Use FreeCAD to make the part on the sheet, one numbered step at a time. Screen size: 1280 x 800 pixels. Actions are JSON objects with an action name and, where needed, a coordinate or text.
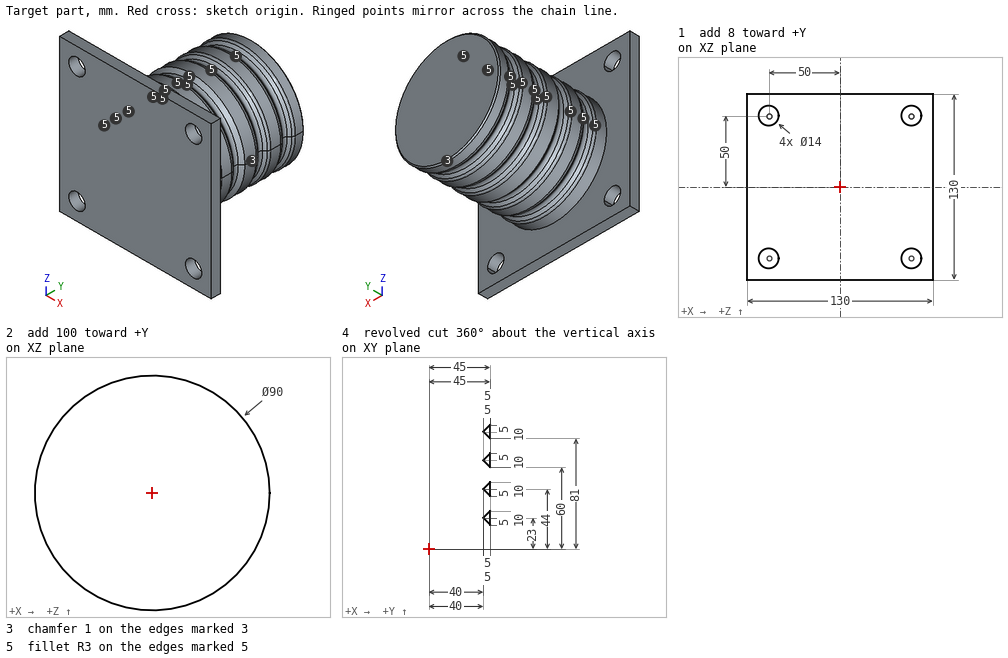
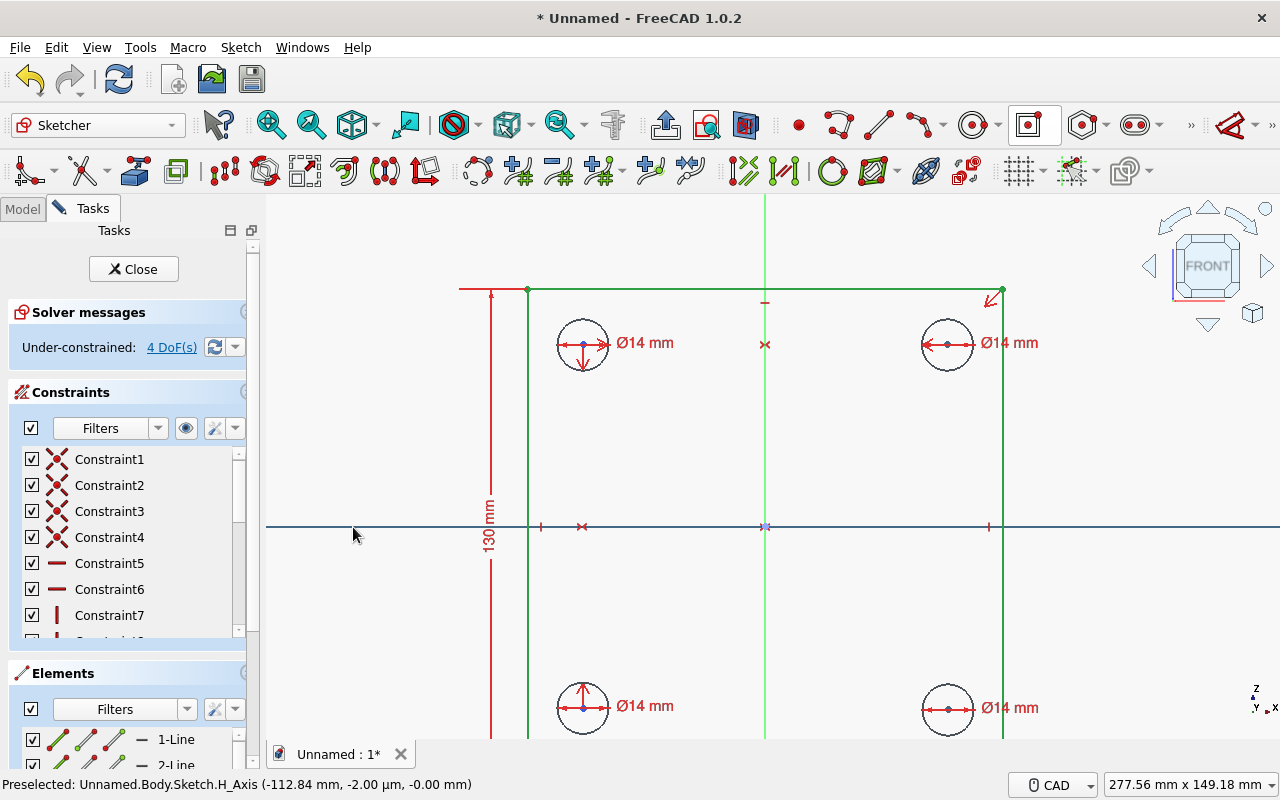
{"action": "key", "text": "s"}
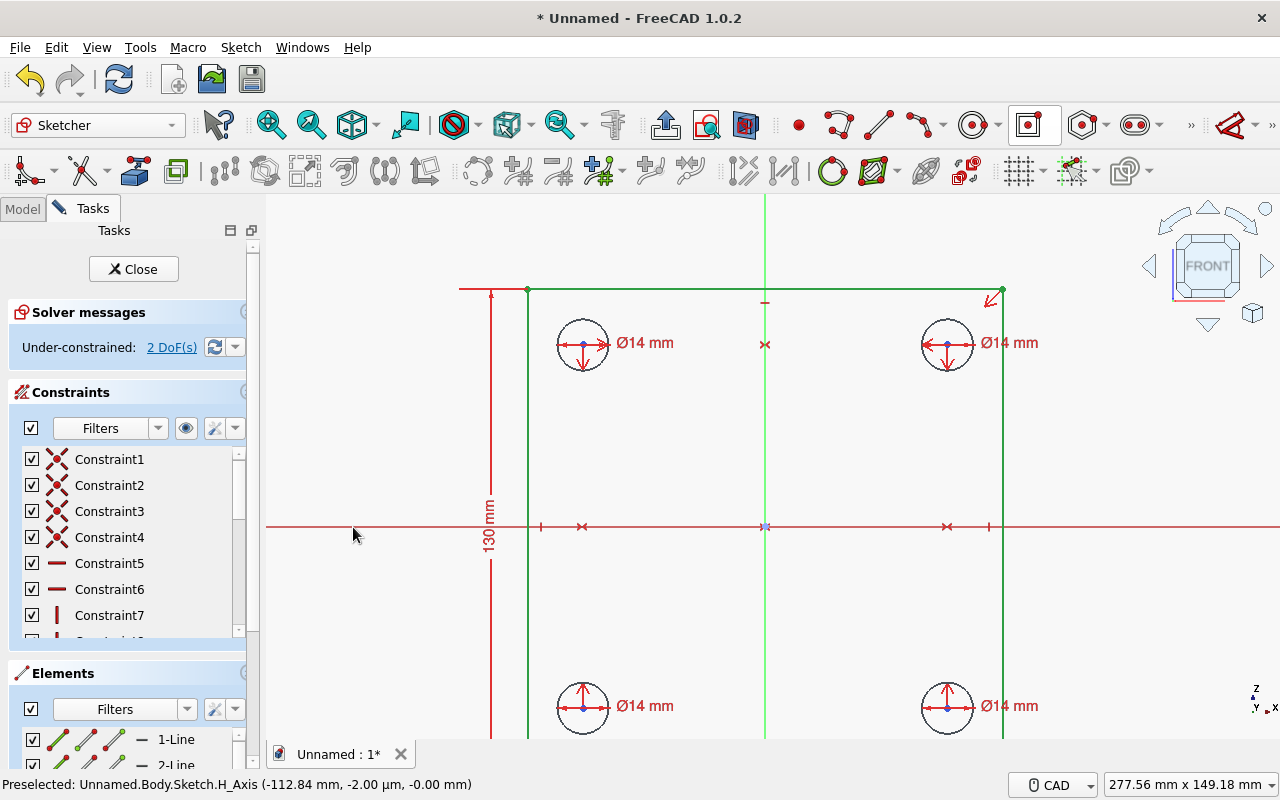
{"action": "left_click", "coordinate": [583, 345]}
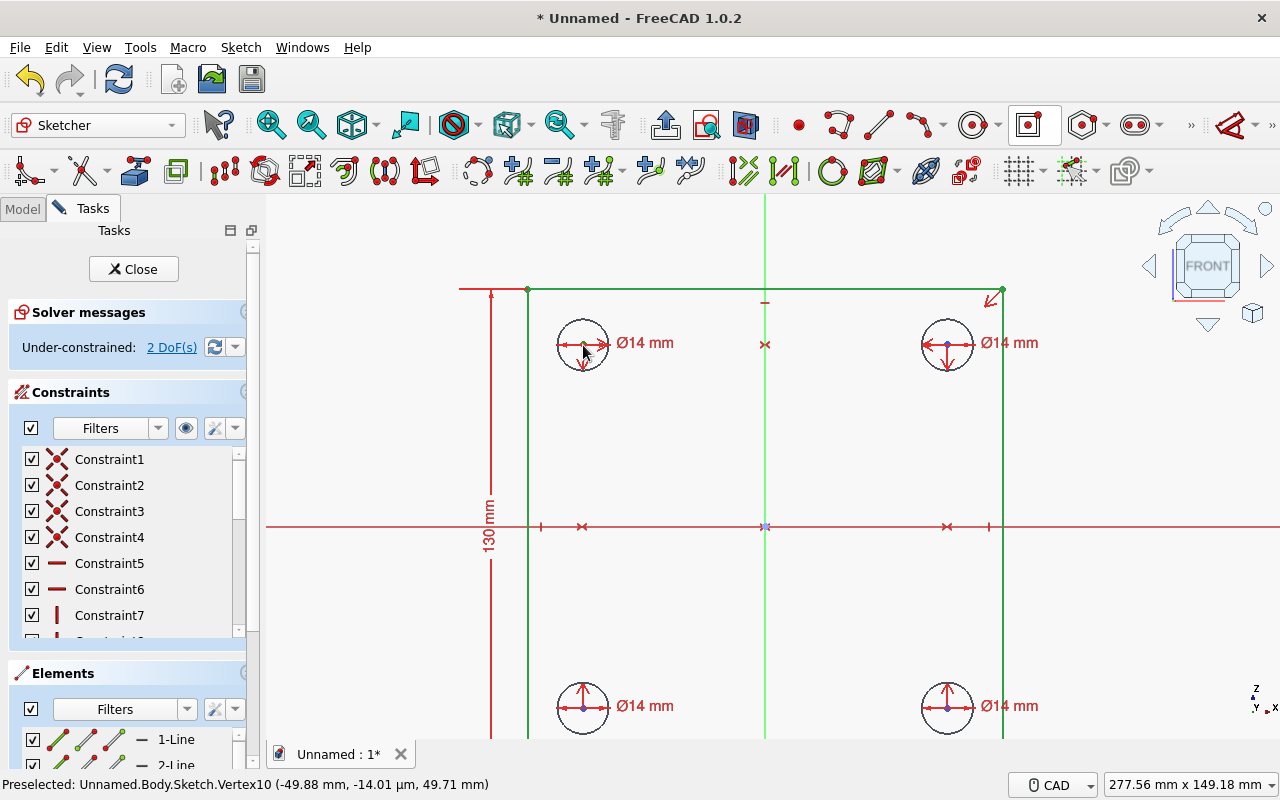
{"action": "left_click", "coordinate": [1258, 126]}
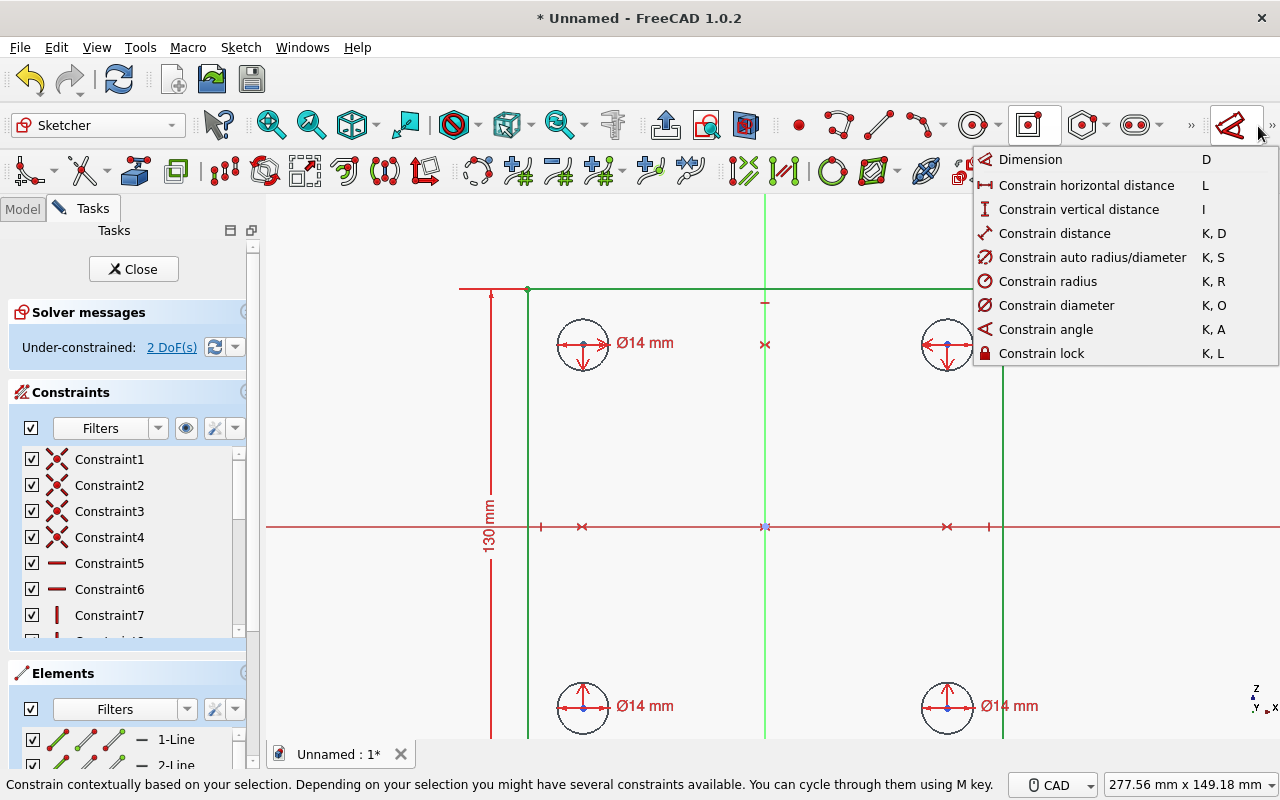
{"action": "left_click", "coordinate": [1126, 185]}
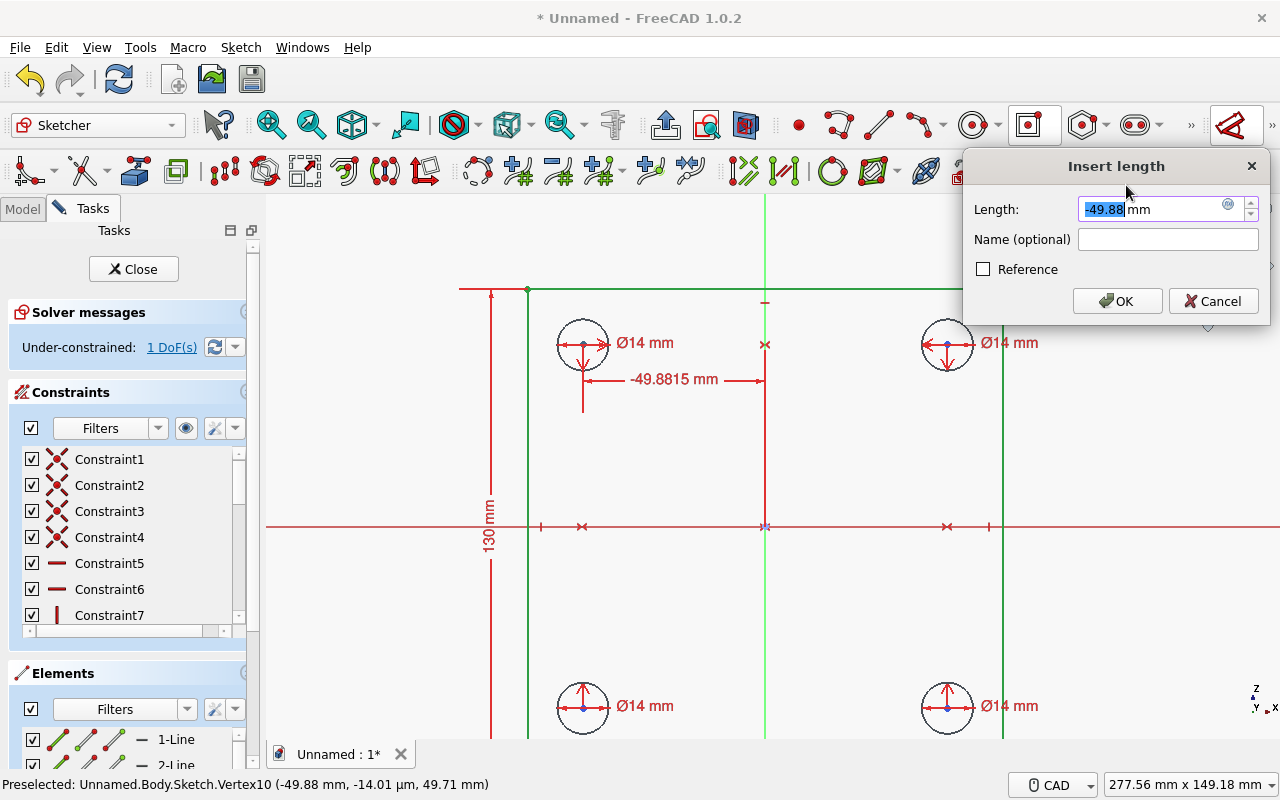
{"action": "type", "text": "-50"}
{"action": "key", "text": "Return"}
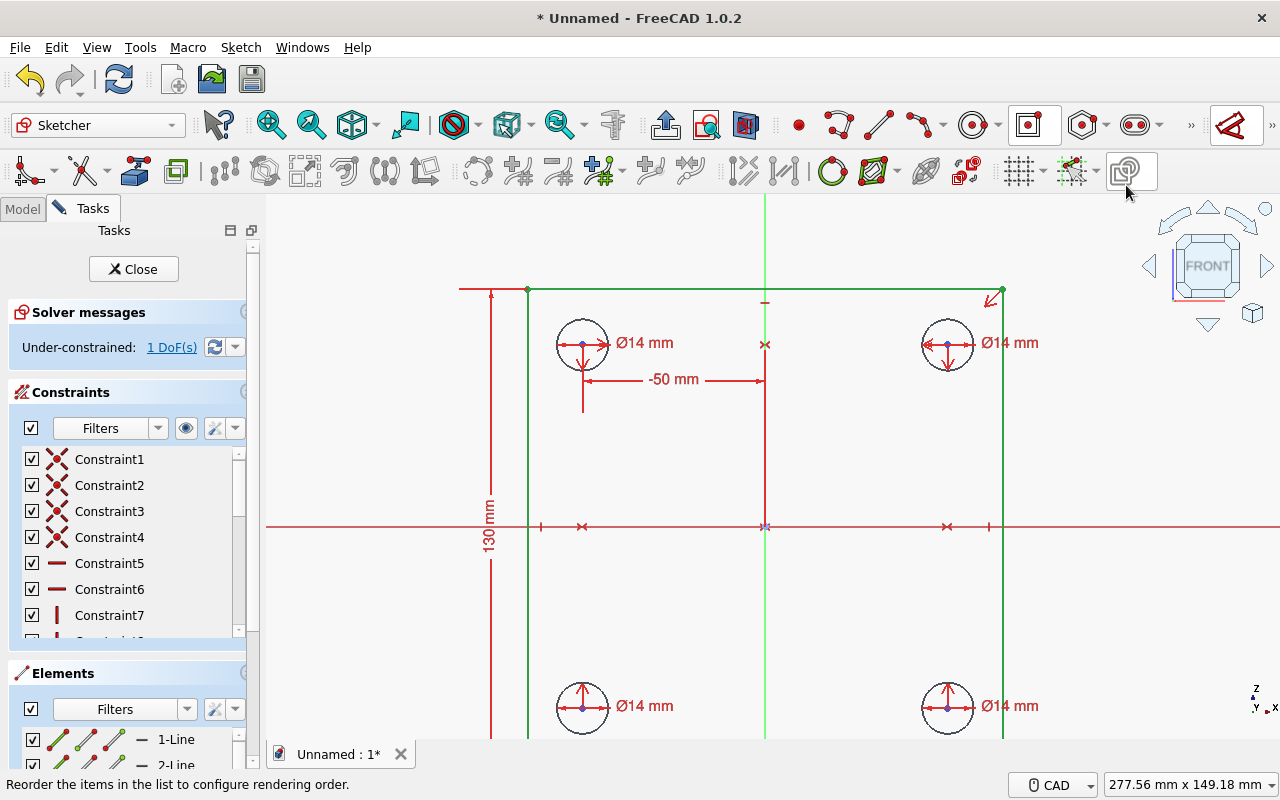
{"action": "left_click", "coordinate": [583, 345]}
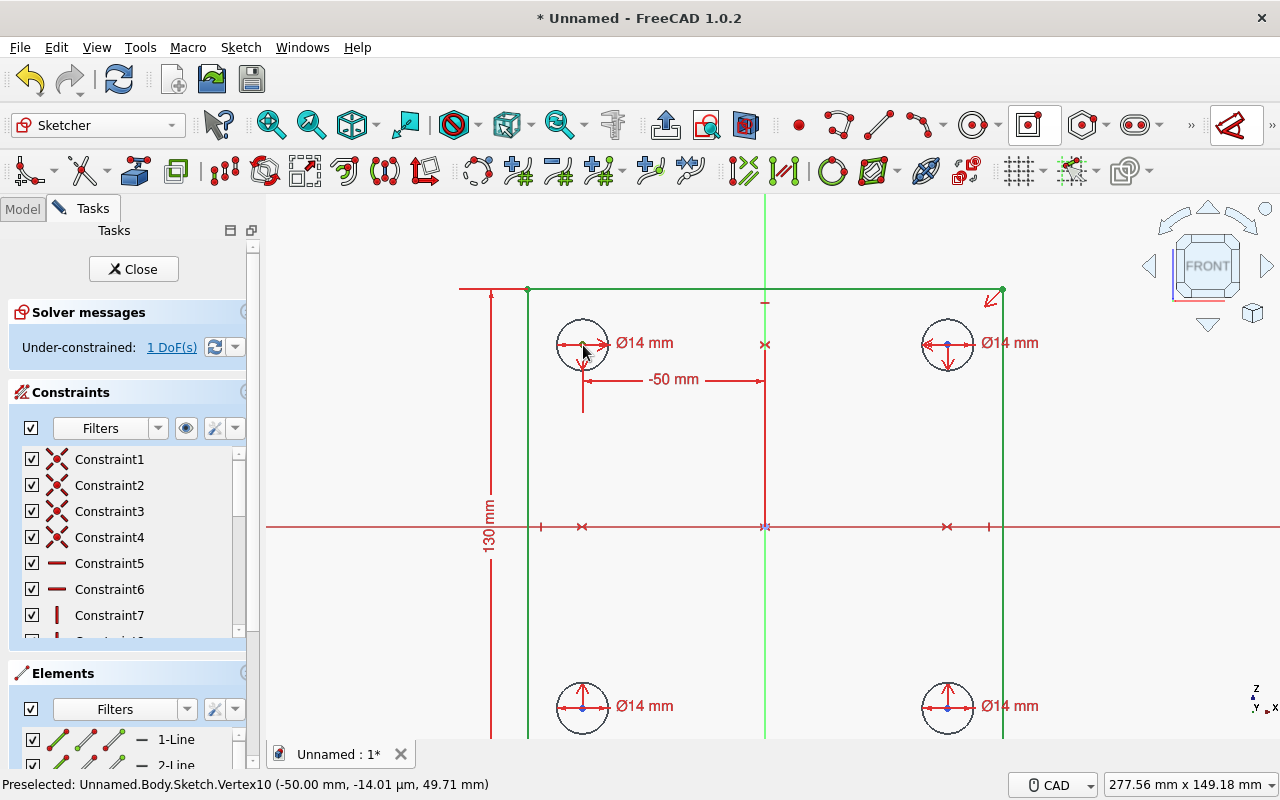
{"action": "left_click", "coordinate": [1258, 126]}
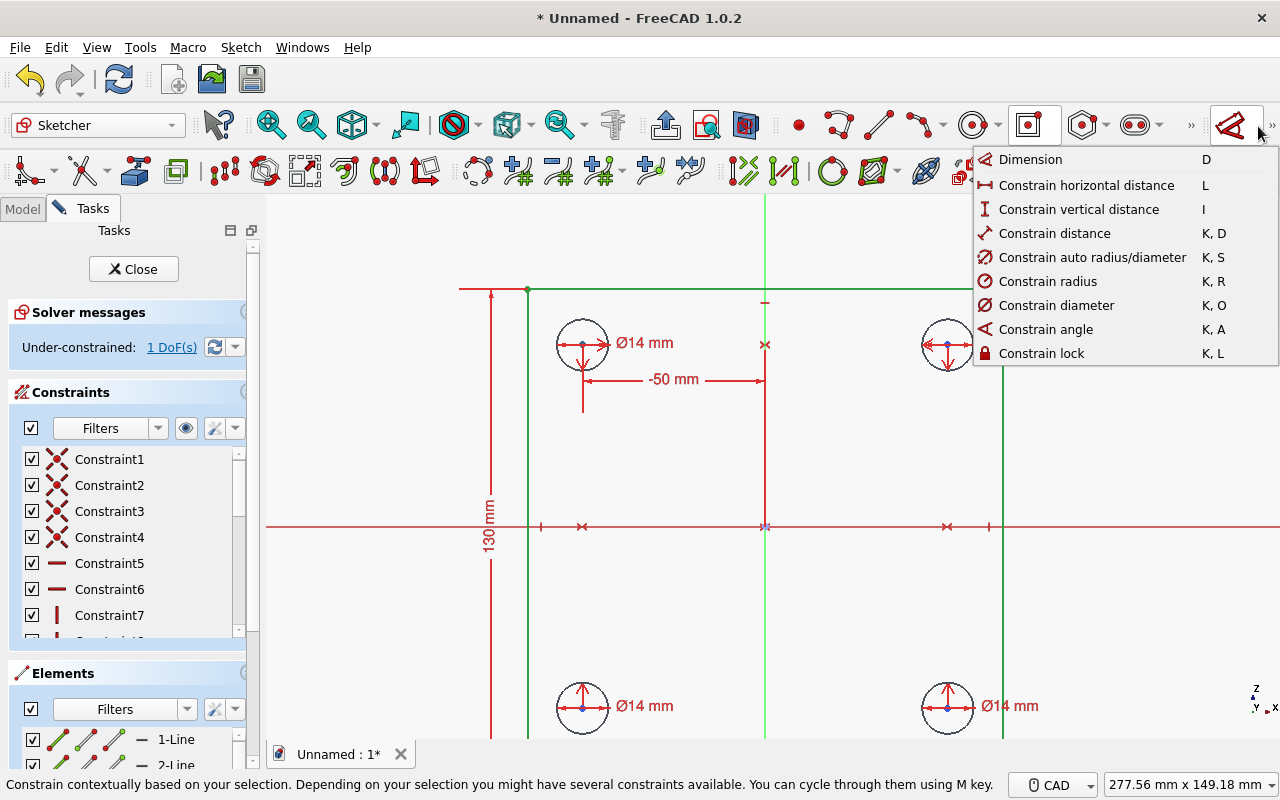
{"action": "left_click", "coordinate": [1126, 209]}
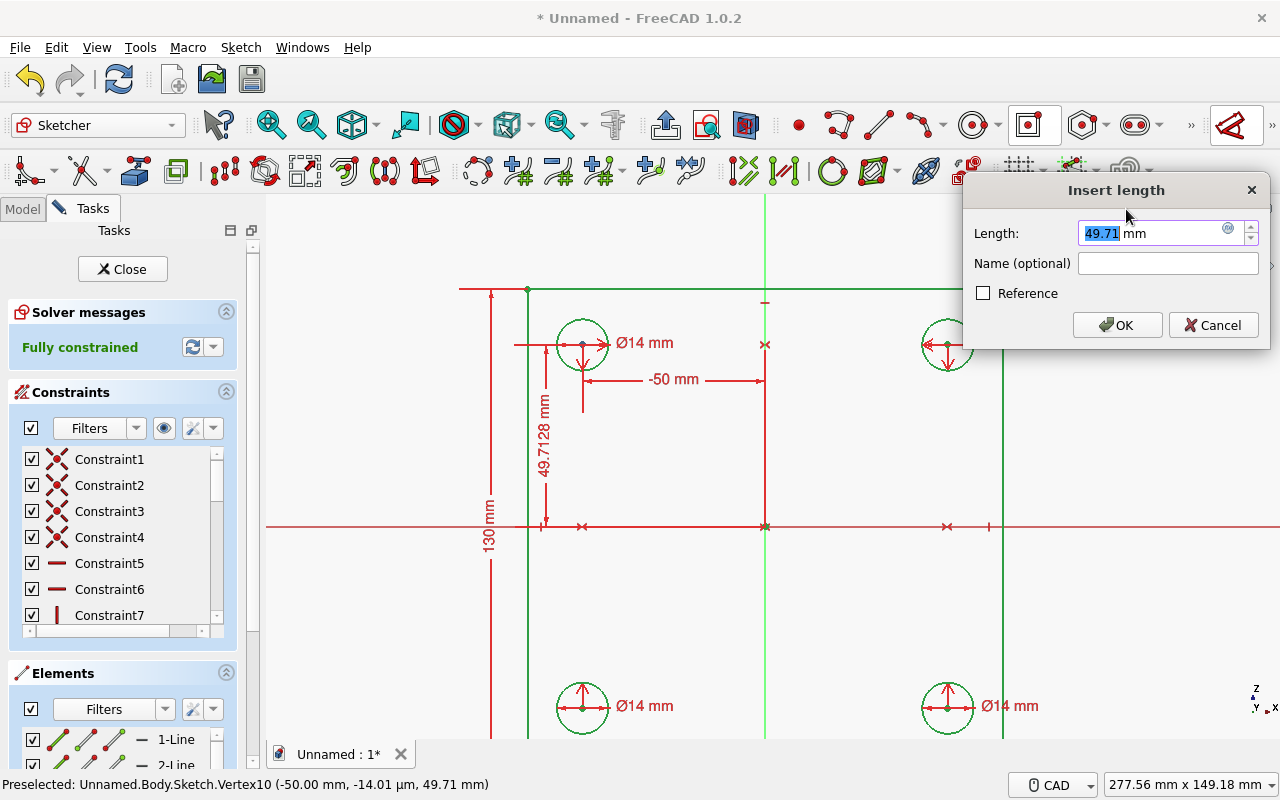
{"action": "type", "text": "50"}
{"action": "key", "text": "Return"}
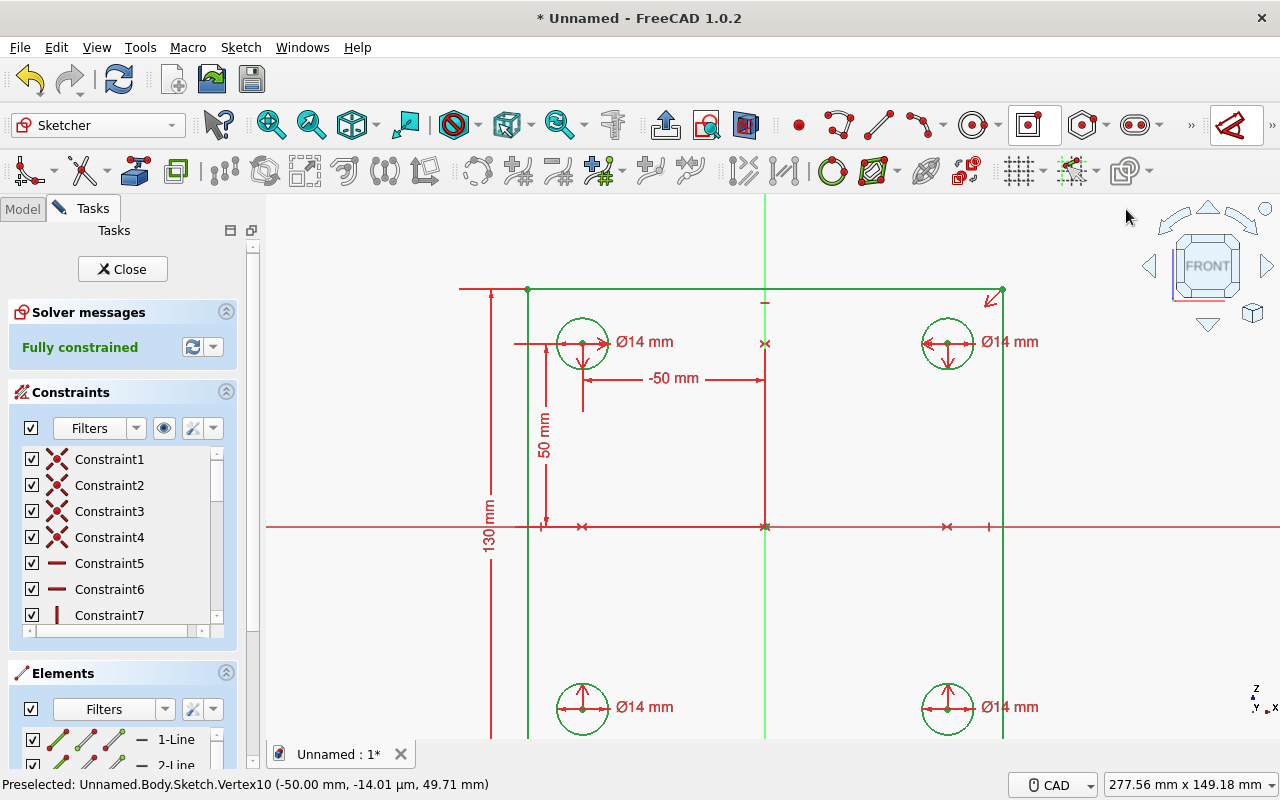
{"action": "left_click", "coordinate": [123, 269]}